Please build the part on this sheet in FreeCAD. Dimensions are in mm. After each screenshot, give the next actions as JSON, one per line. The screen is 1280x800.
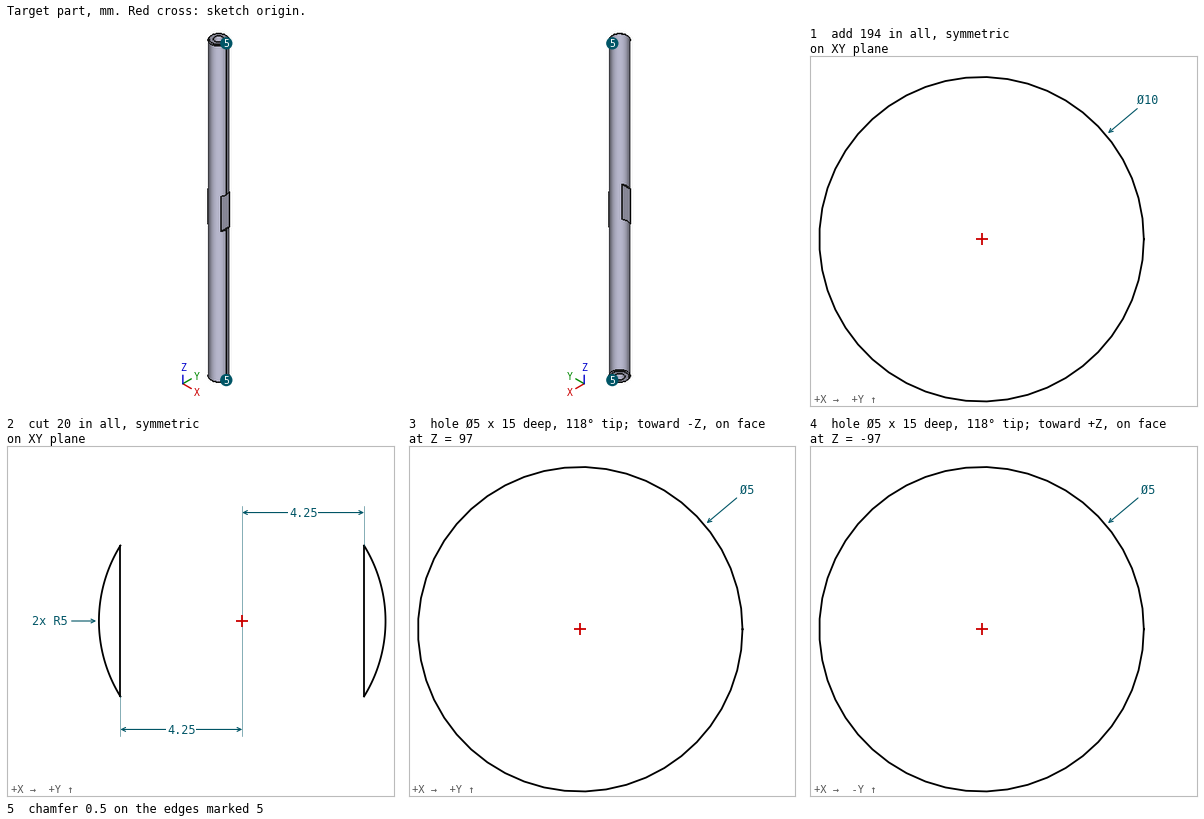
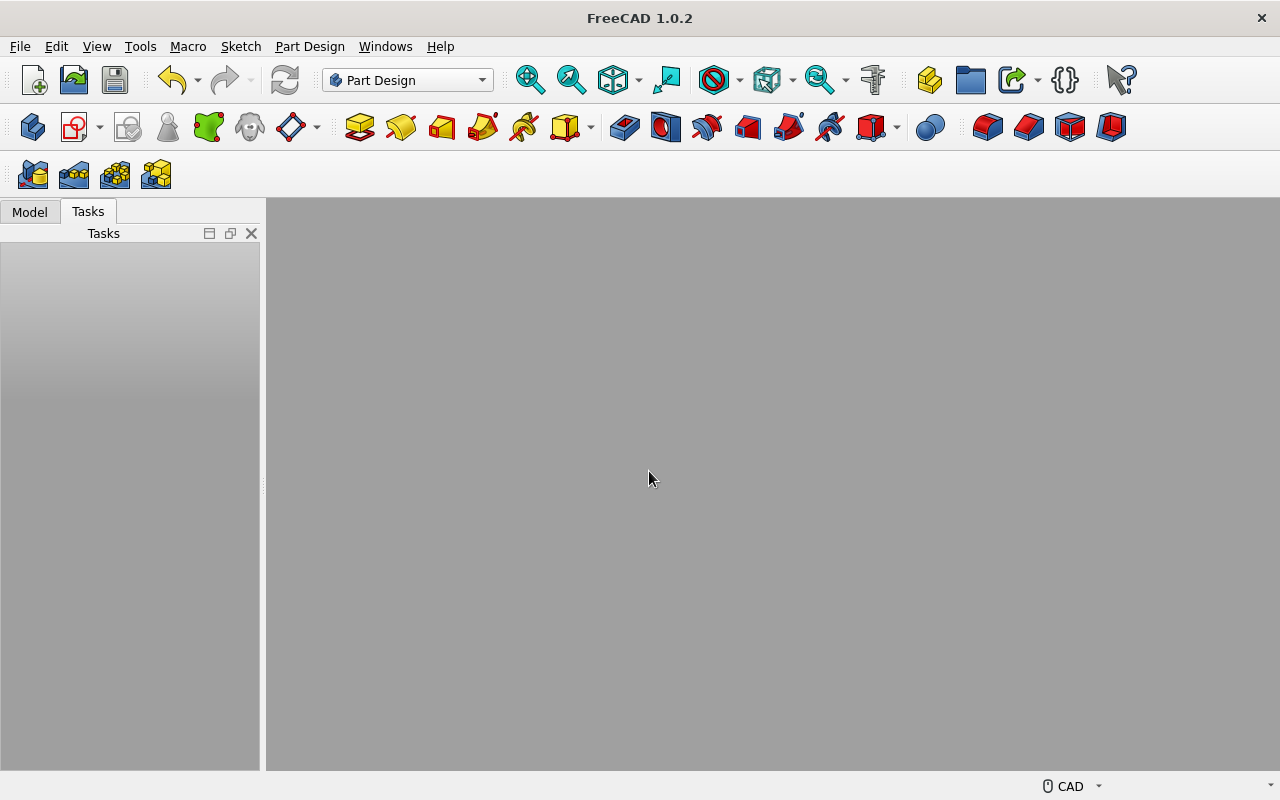
{"action": "left_click", "coordinate": [33, 80]}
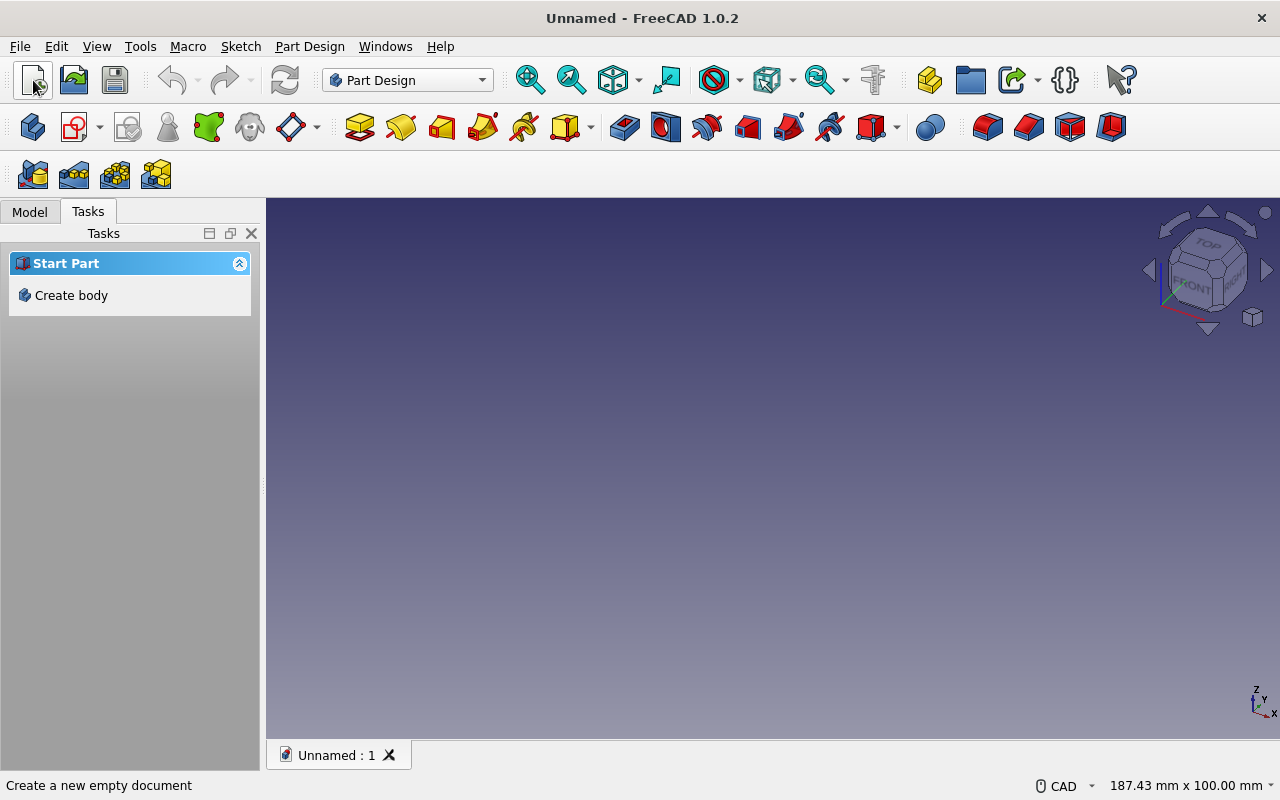
{"action": "left_click", "coordinate": [74, 128]}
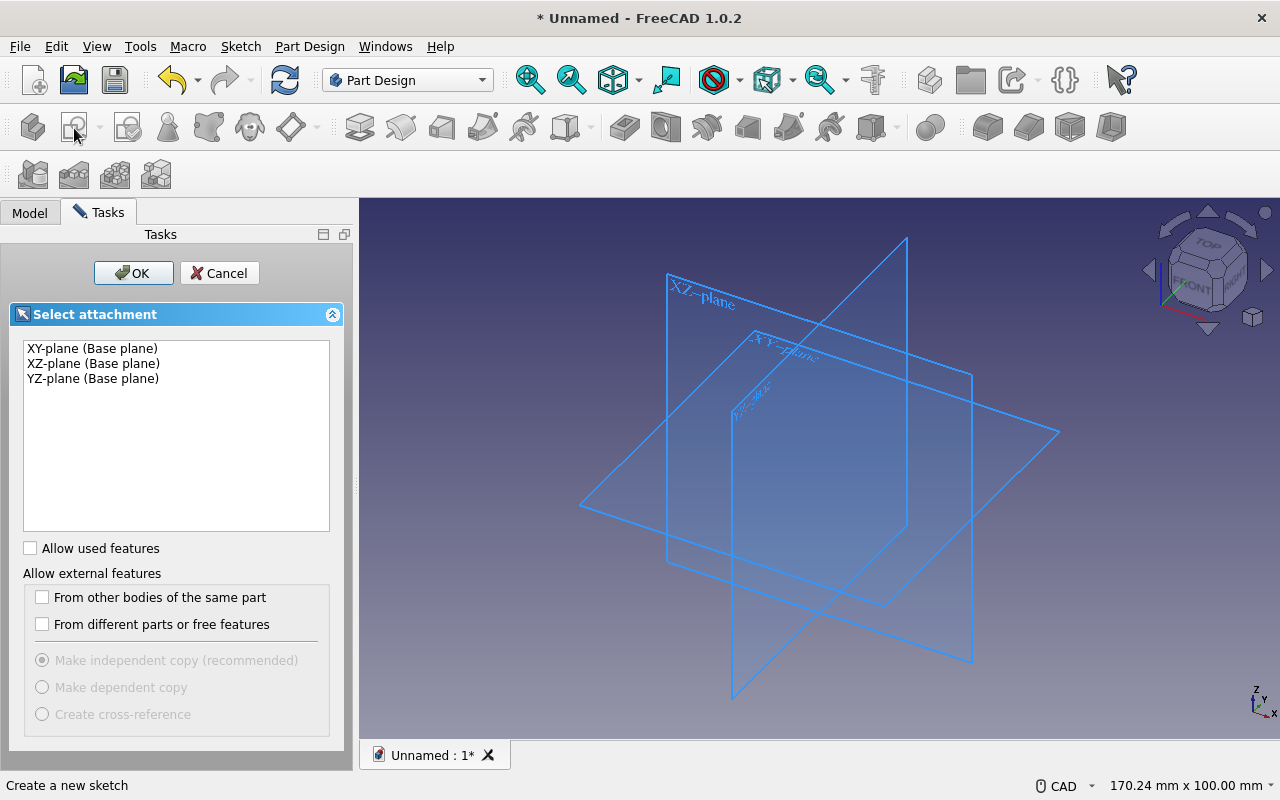
{"action": "left_click", "coordinate": [84, 348]}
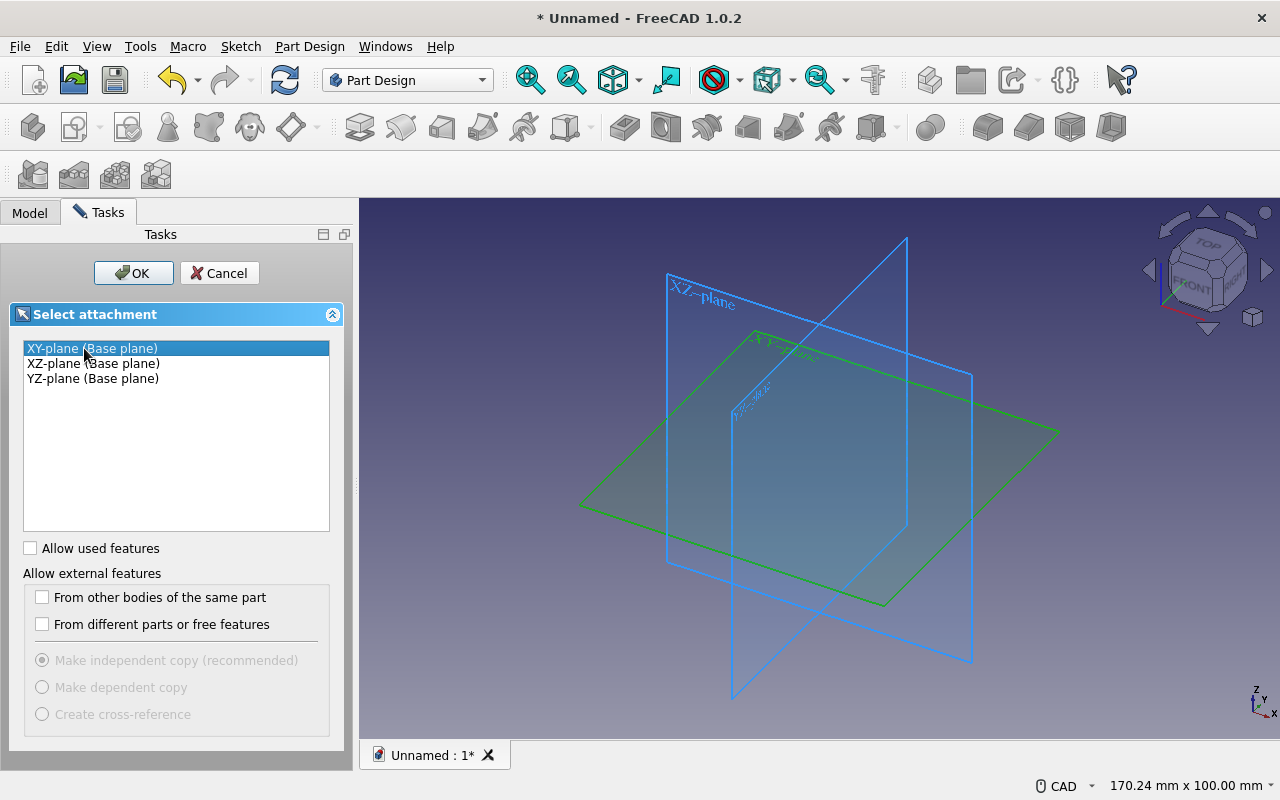
{"action": "left_click", "coordinate": [134, 273]}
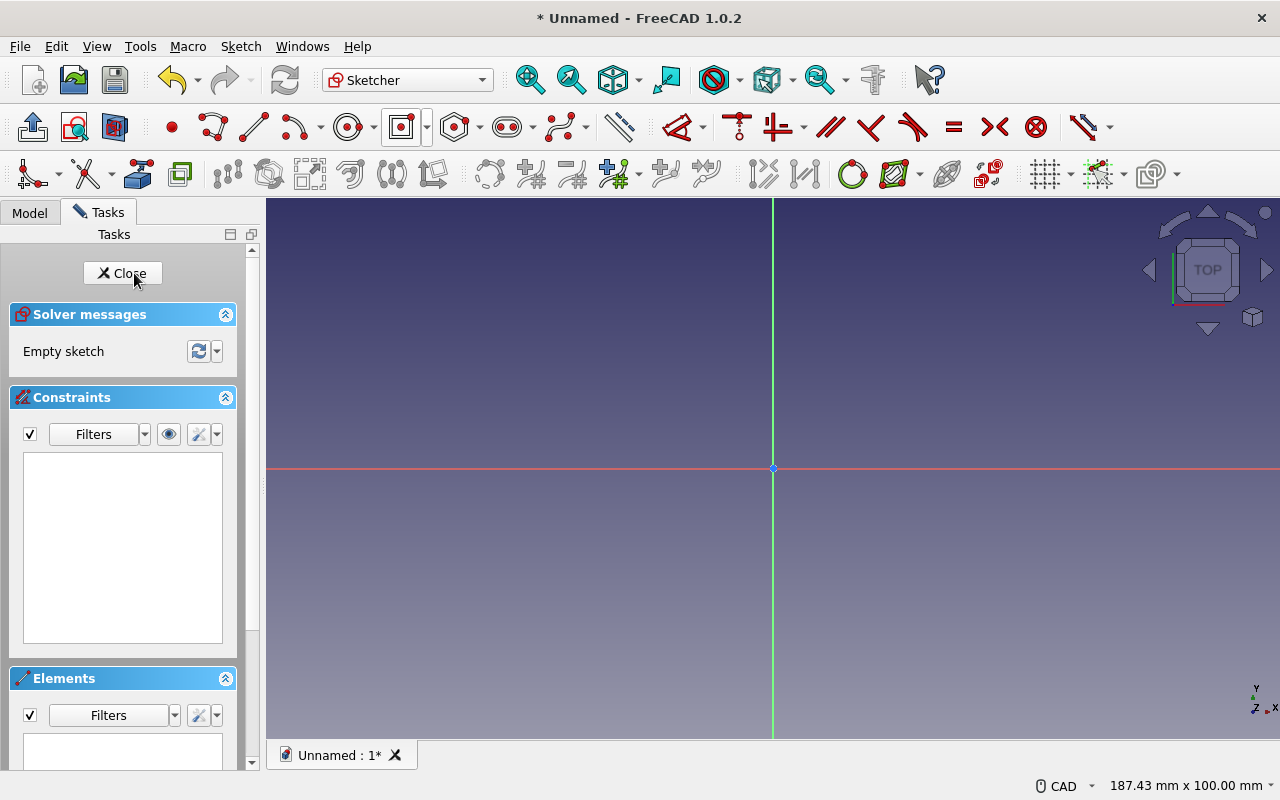
{"action": "scroll", "coordinate": [787, 468], "scroll_direction": "up", "scroll_amount": 9}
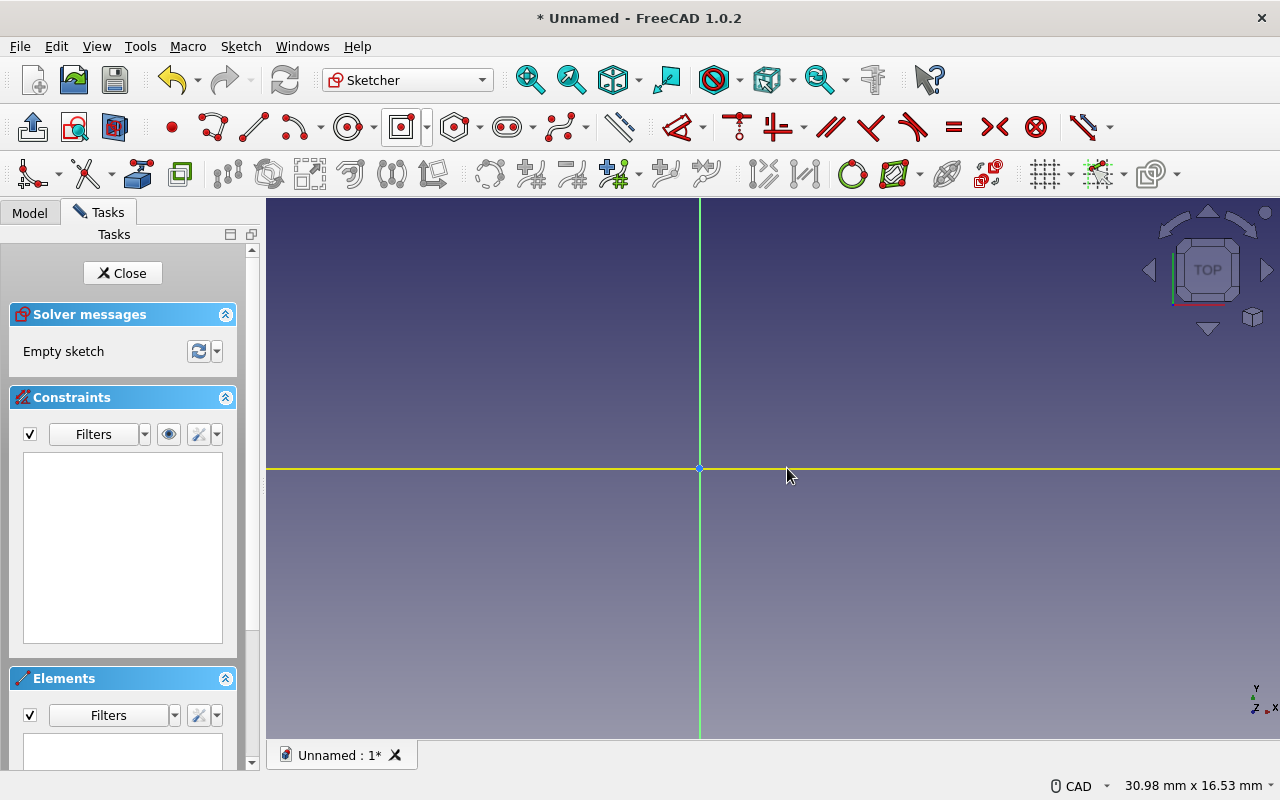
{"action": "left_click", "coordinate": [348, 128]}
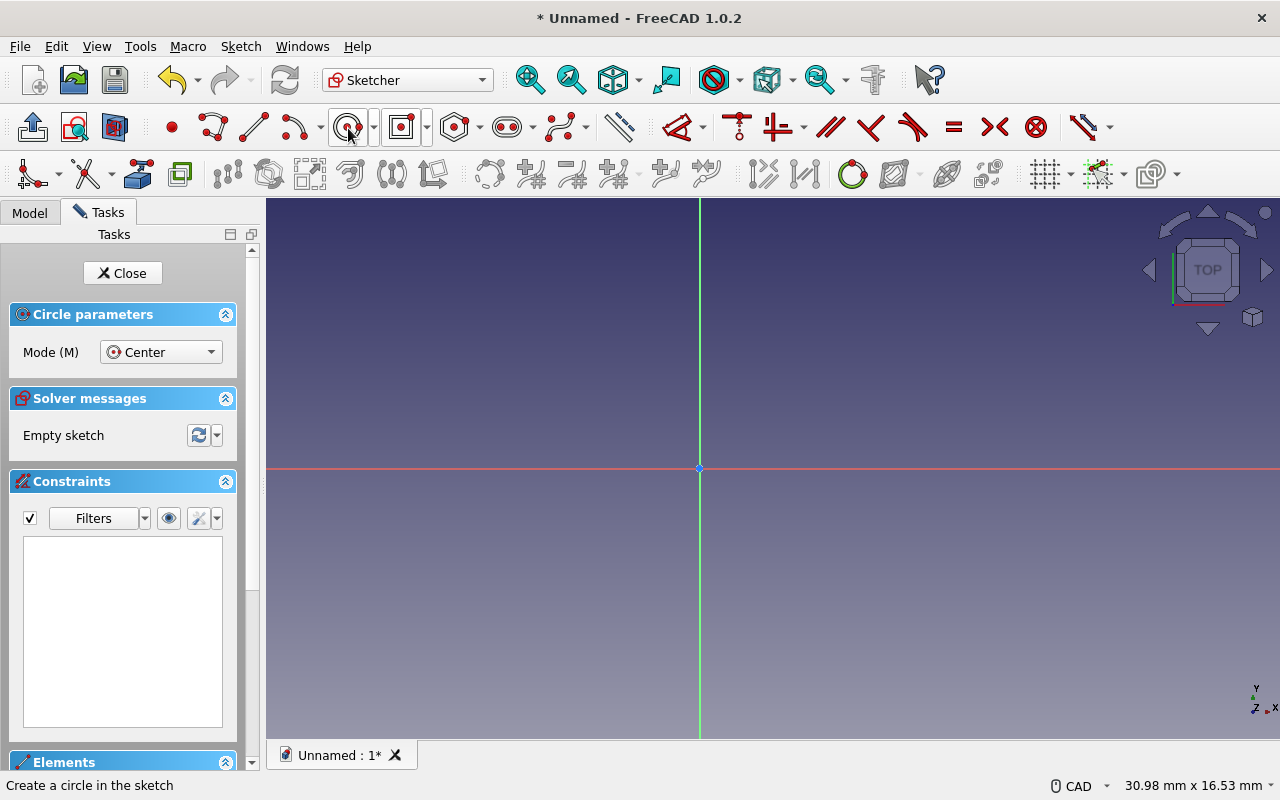
{"action": "left_click", "coordinate": [700, 468]}
{"action": "left_click", "coordinate": [815, 353]}
{"action": "key", "text": "Escape"}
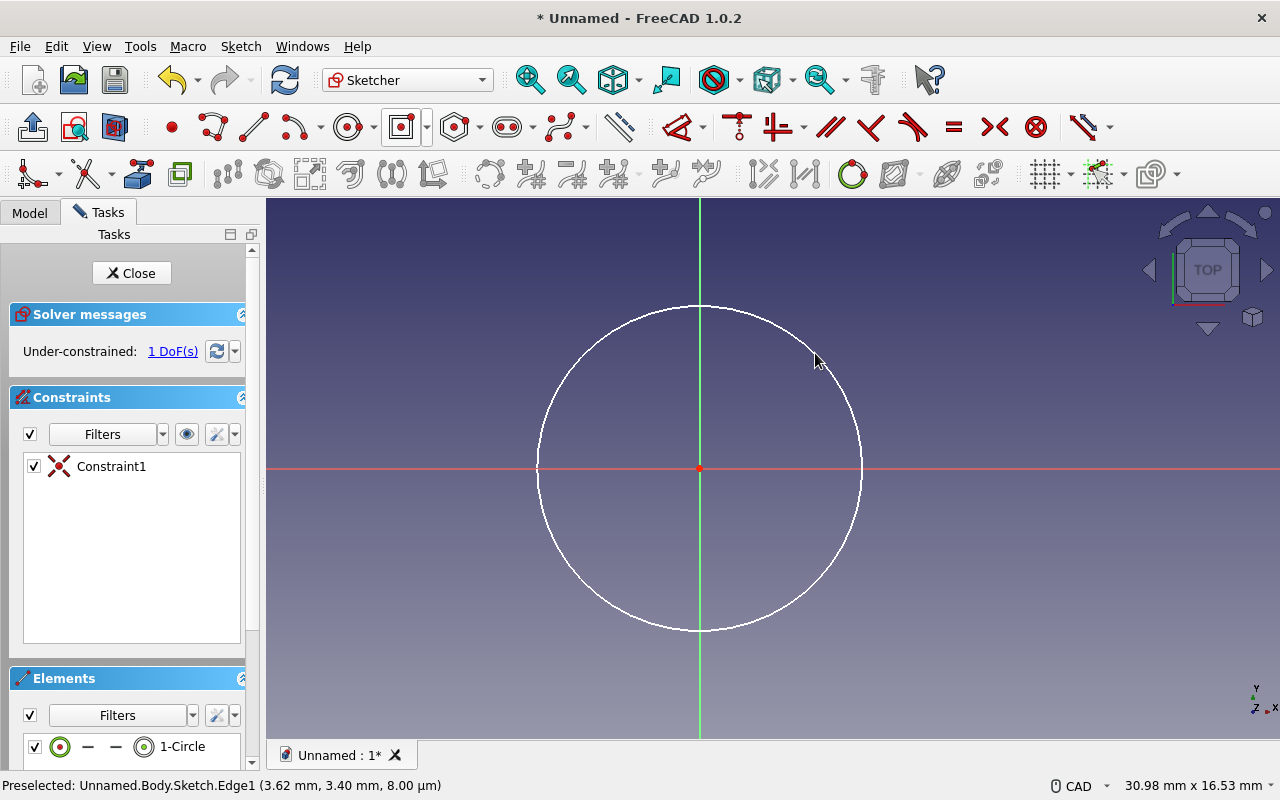
{"action": "left_click", "coordinate": [814, 353]}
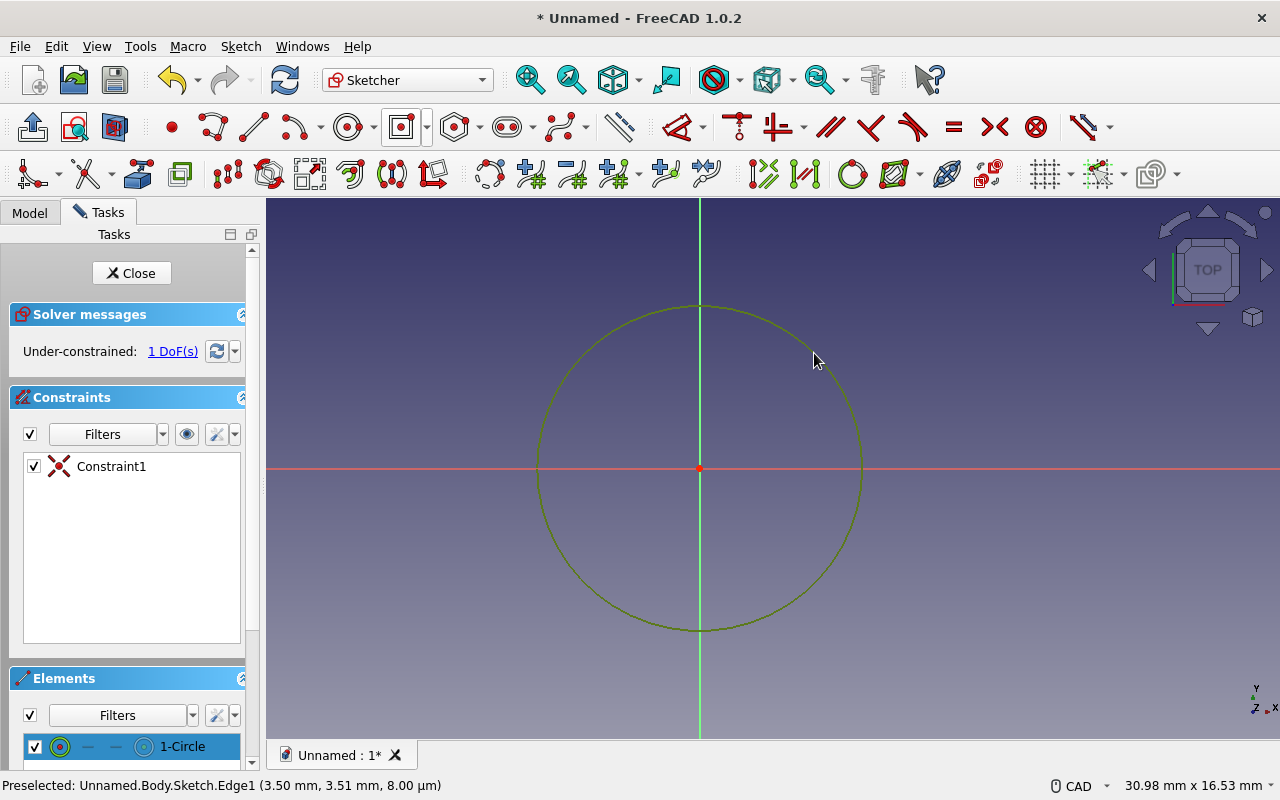
{"action": "left_click", "coordinate": [702, 128]}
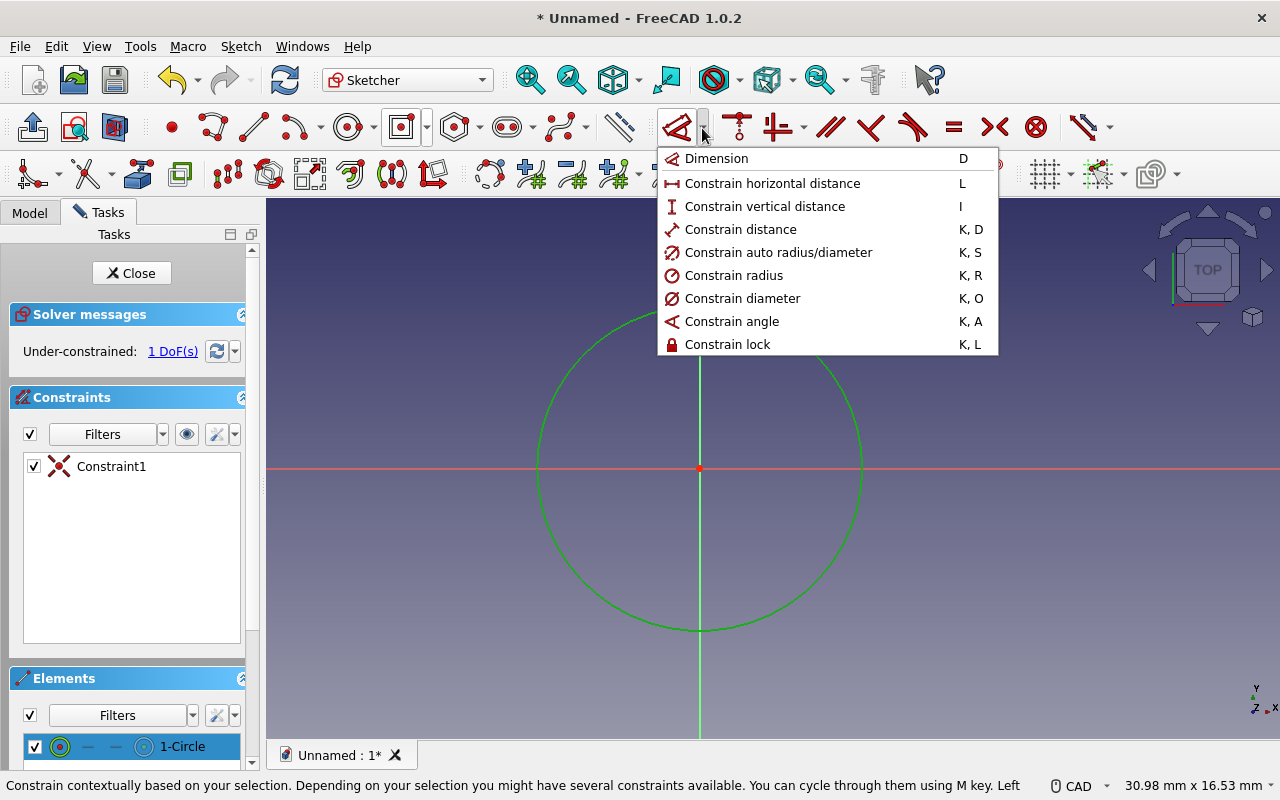
{"action": "left_click", "coordinate": [828, 298]}